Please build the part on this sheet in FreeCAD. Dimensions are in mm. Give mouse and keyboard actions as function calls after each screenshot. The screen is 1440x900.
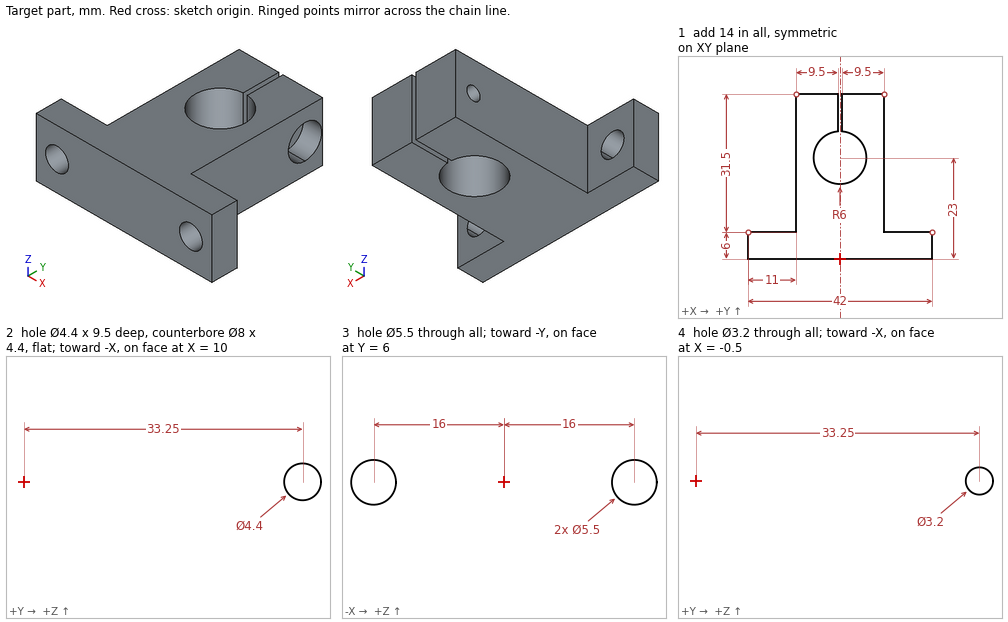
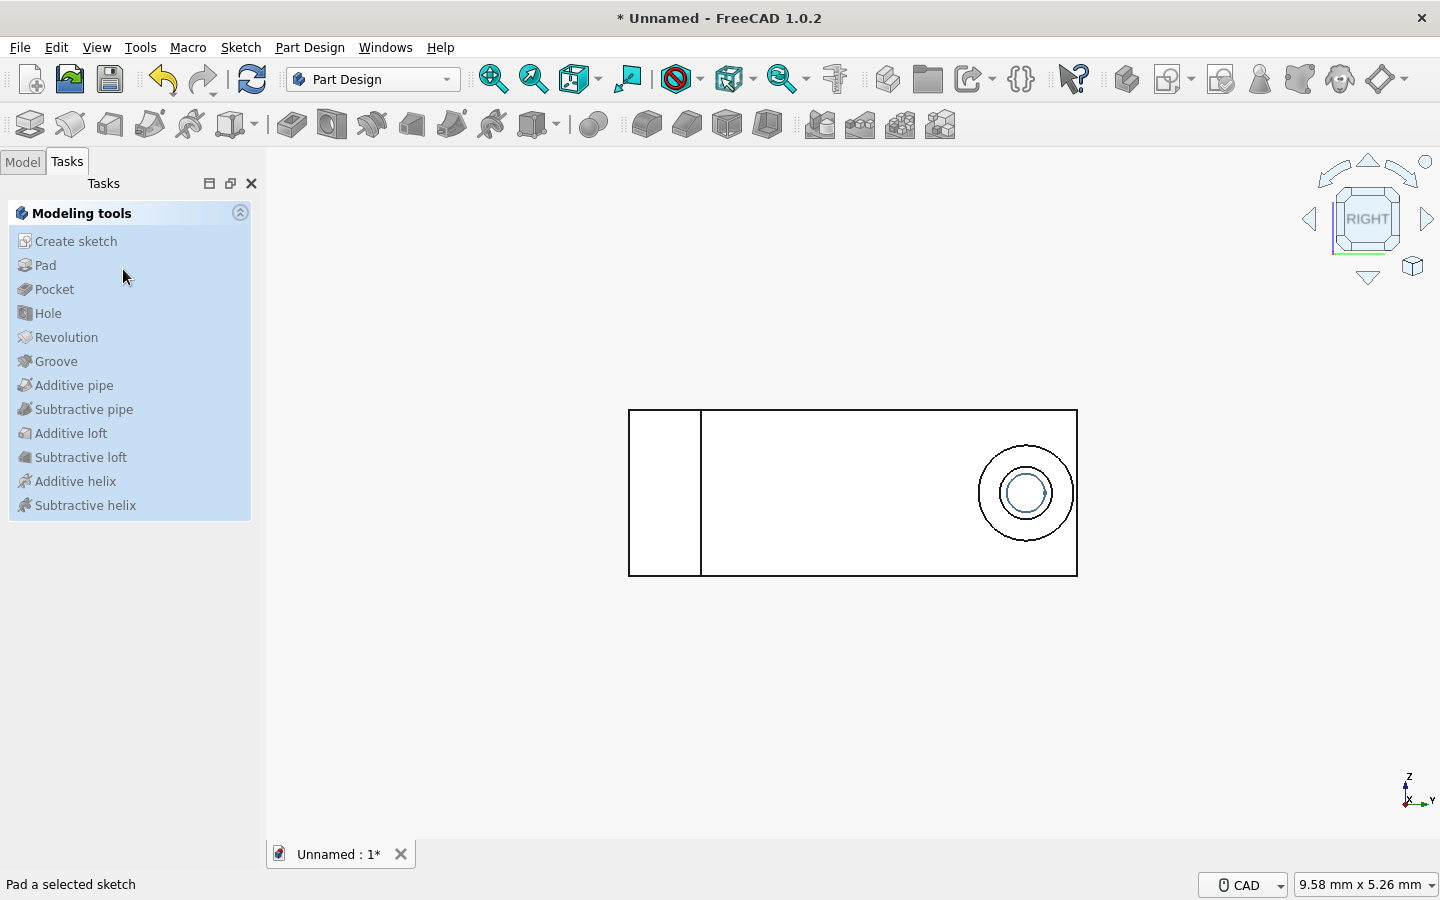
click(332, 124)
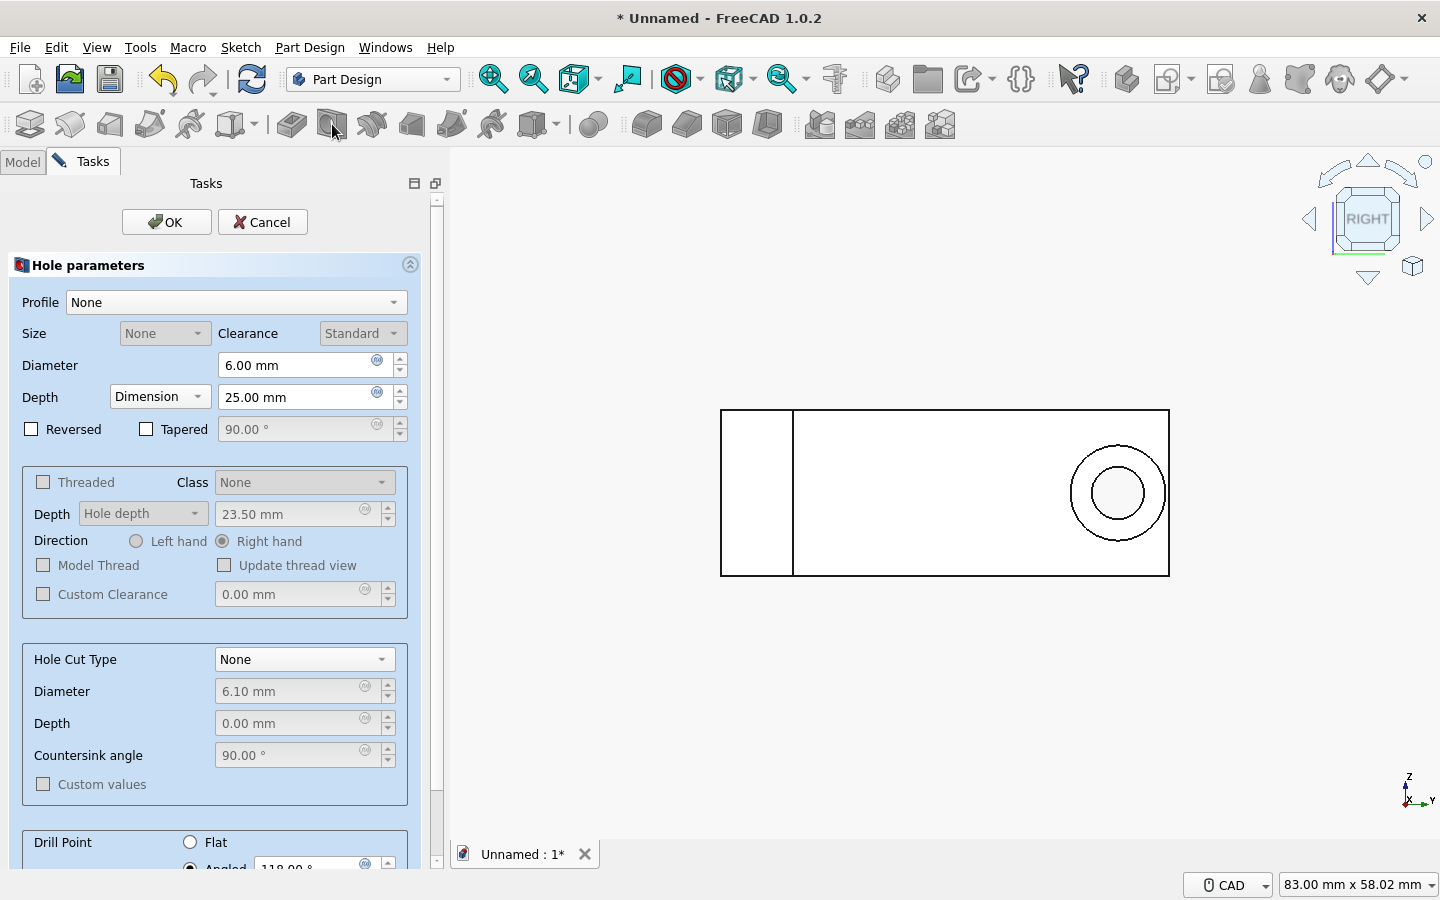
triple_click(305, 365)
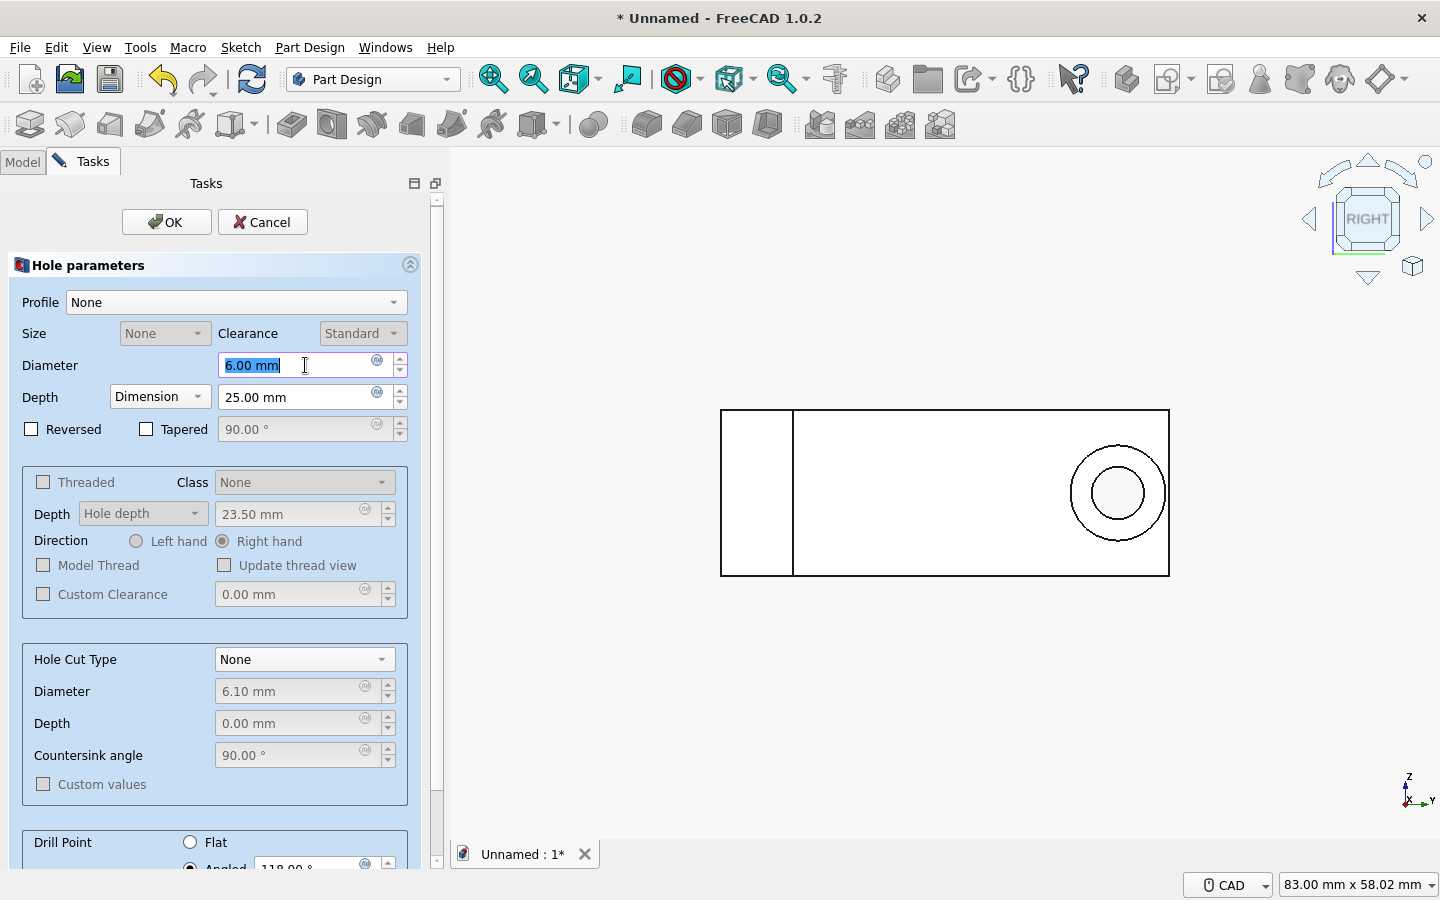
text(3.2)
key(Tab)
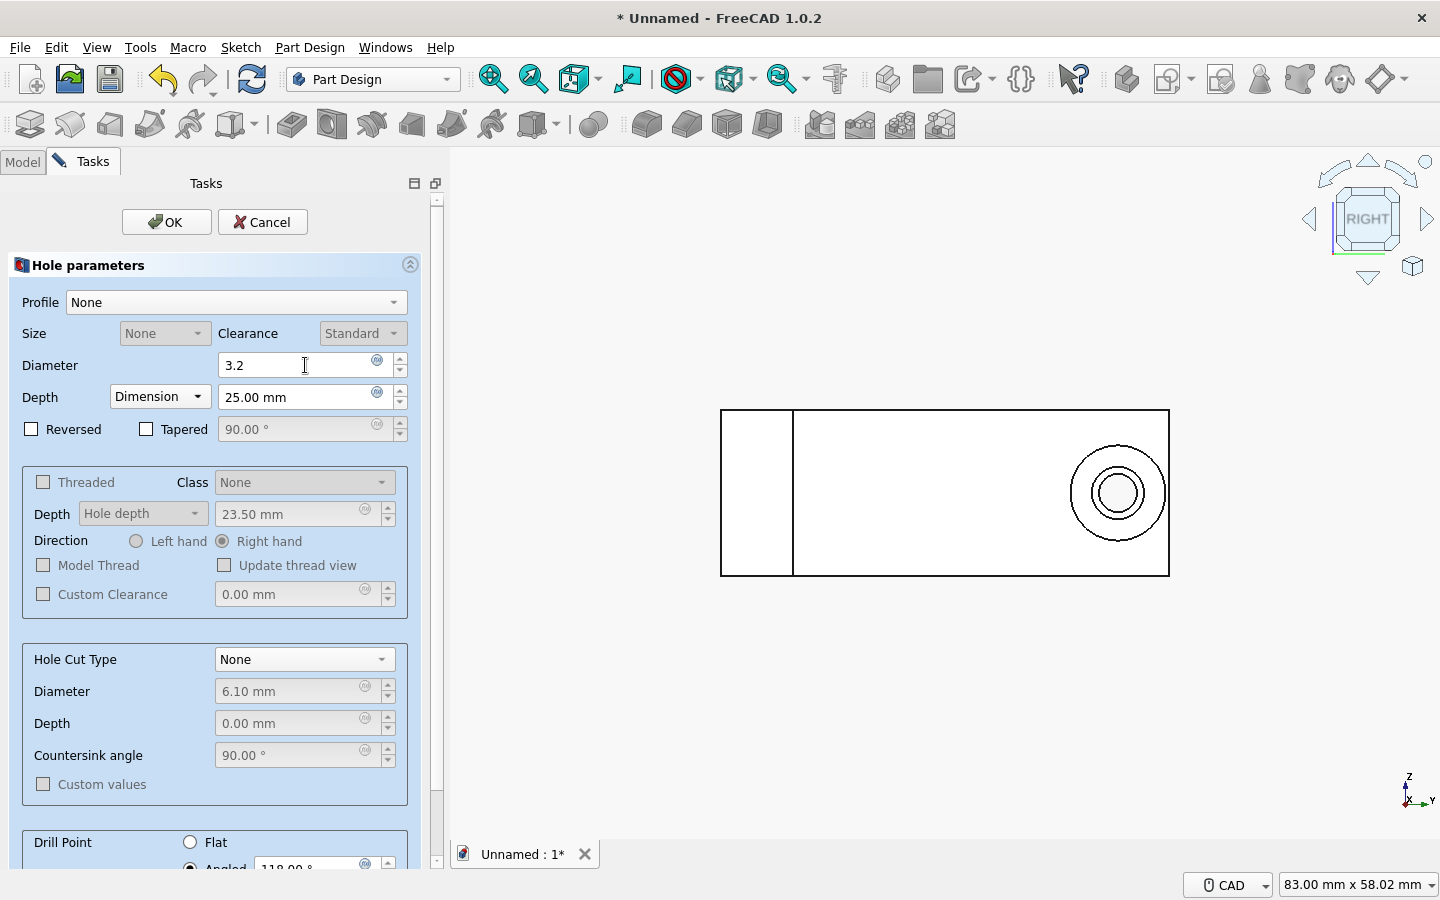
click(161, 396)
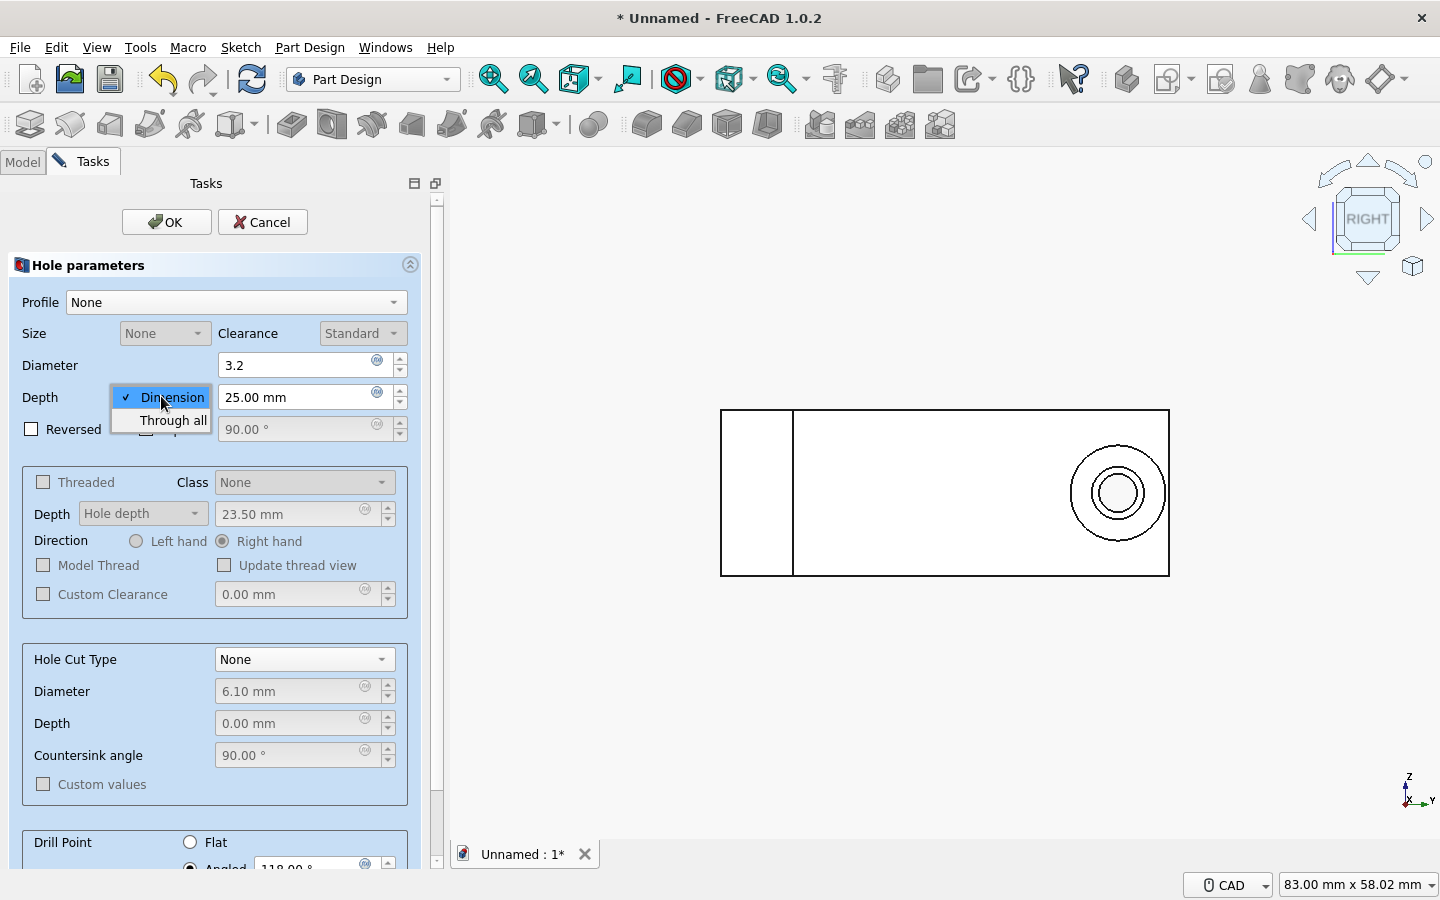
click(160, 420)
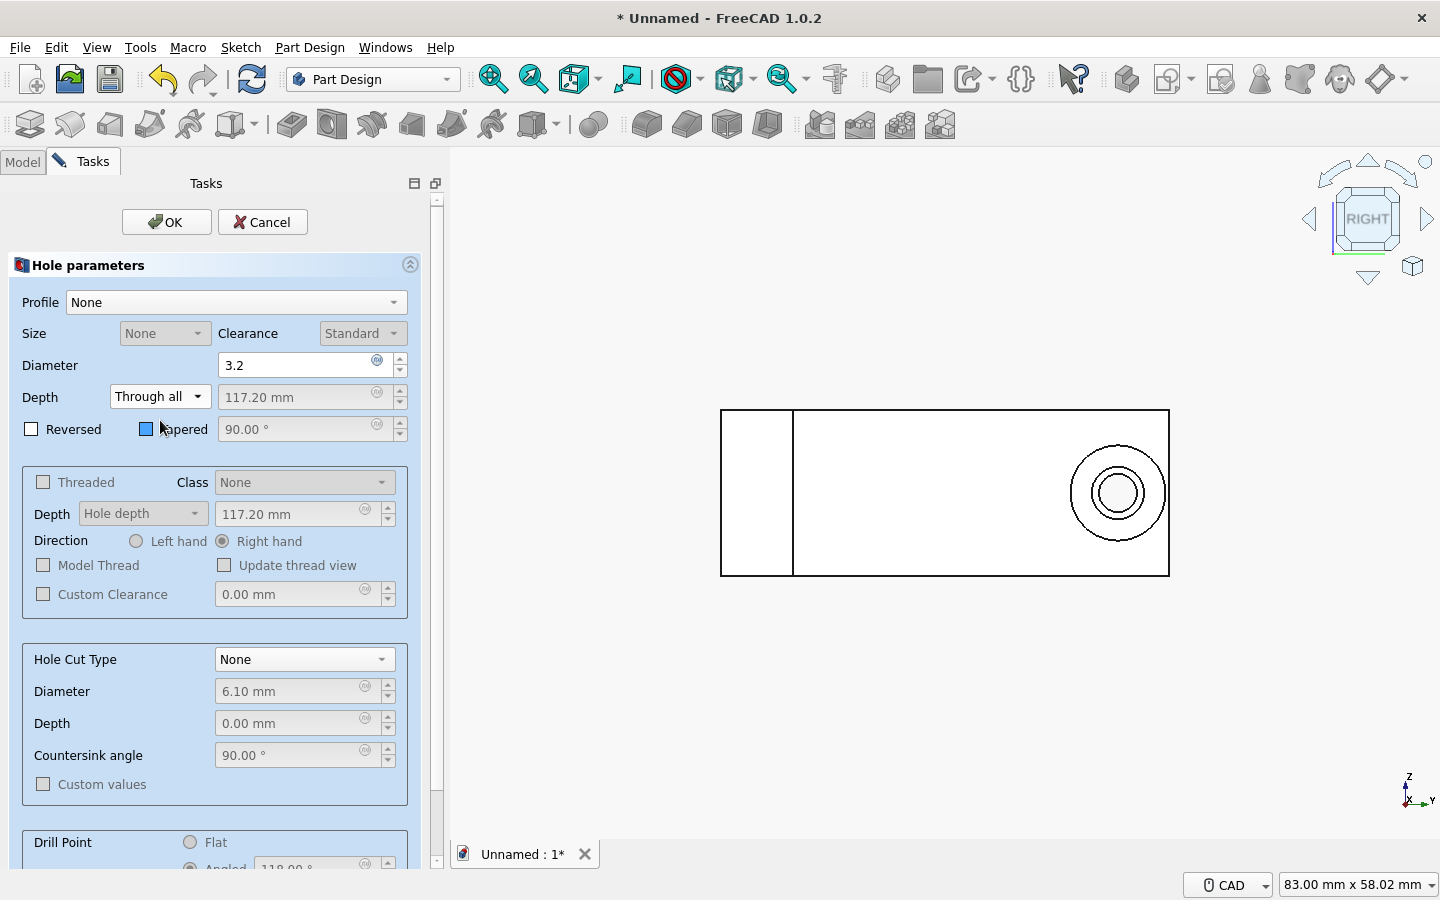
click(167, 222)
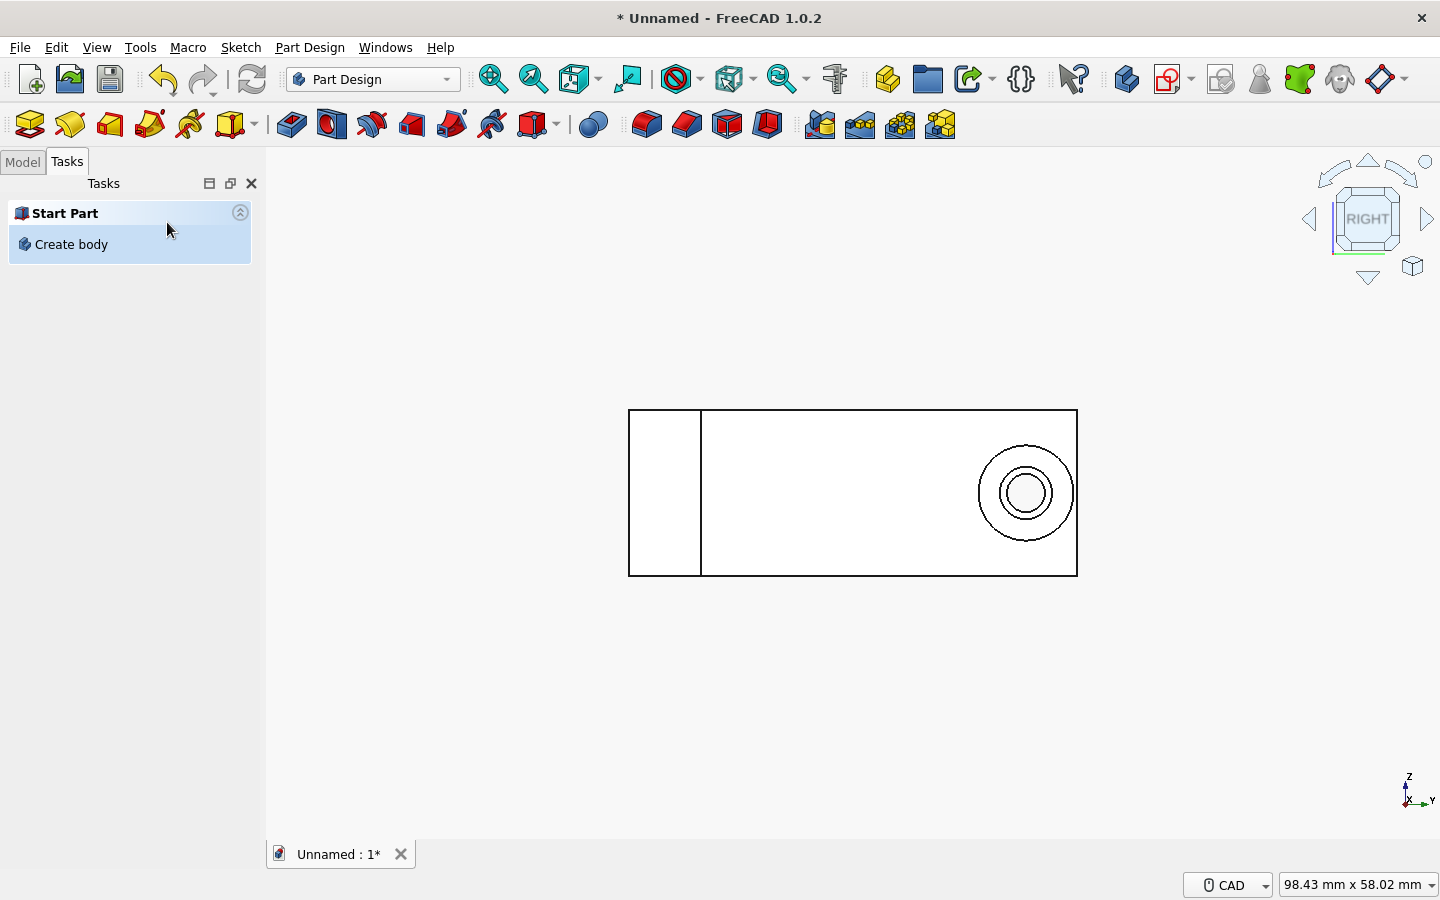
key(0)